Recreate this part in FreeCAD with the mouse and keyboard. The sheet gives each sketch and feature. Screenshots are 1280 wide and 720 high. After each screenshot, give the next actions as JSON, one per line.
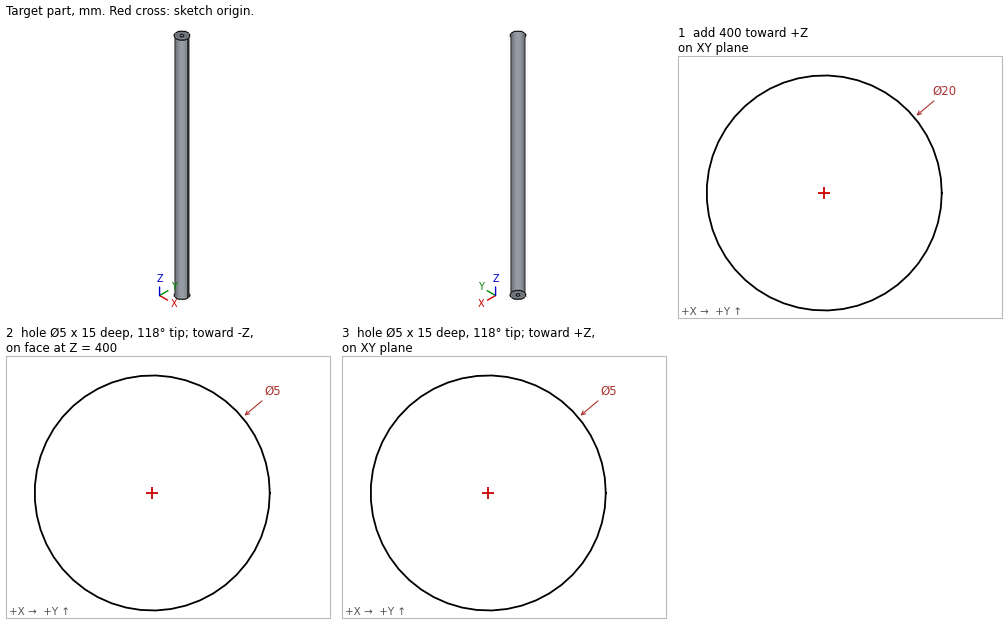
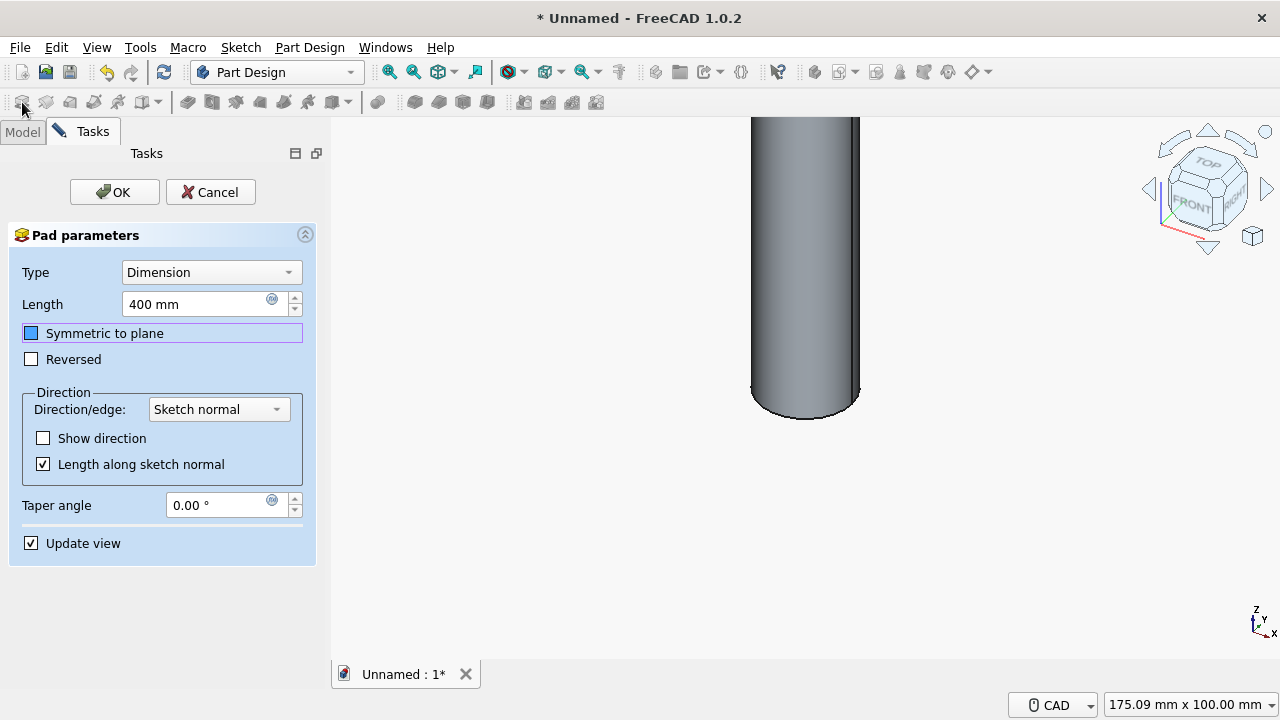
{"action": "left_click", "coordinate": [115, 192]}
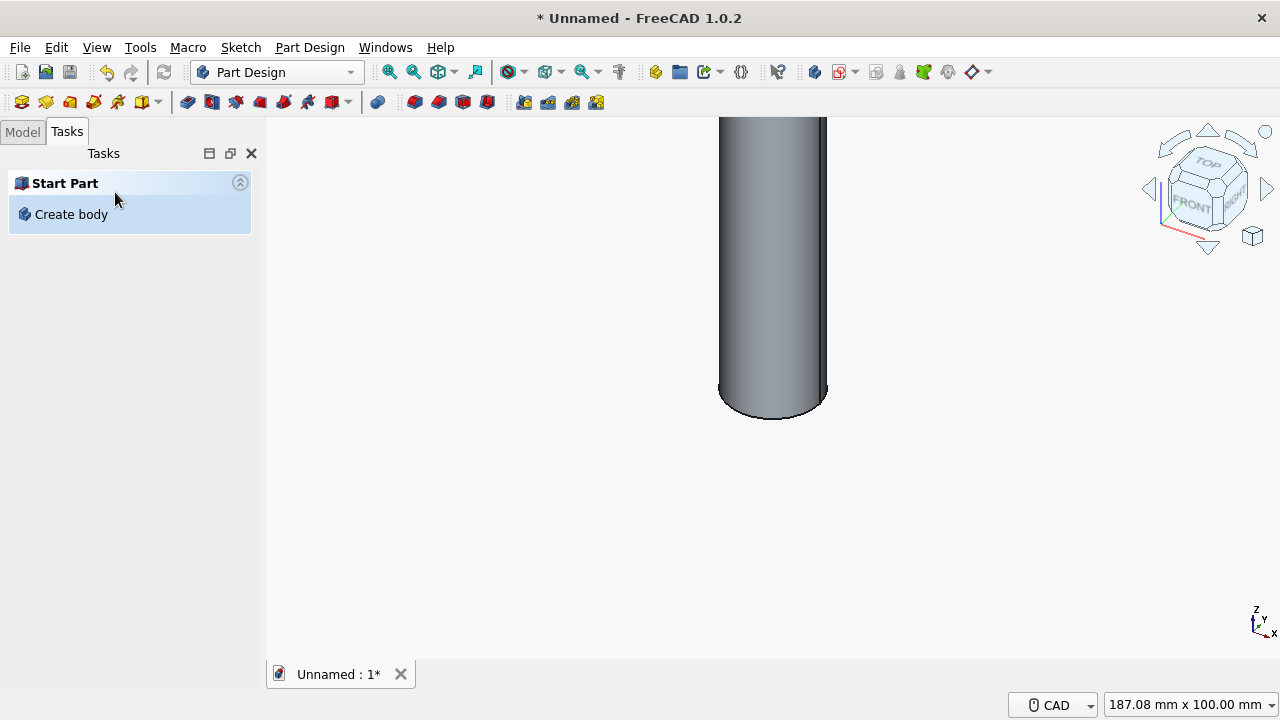
{"action": "key", "text": "v f"}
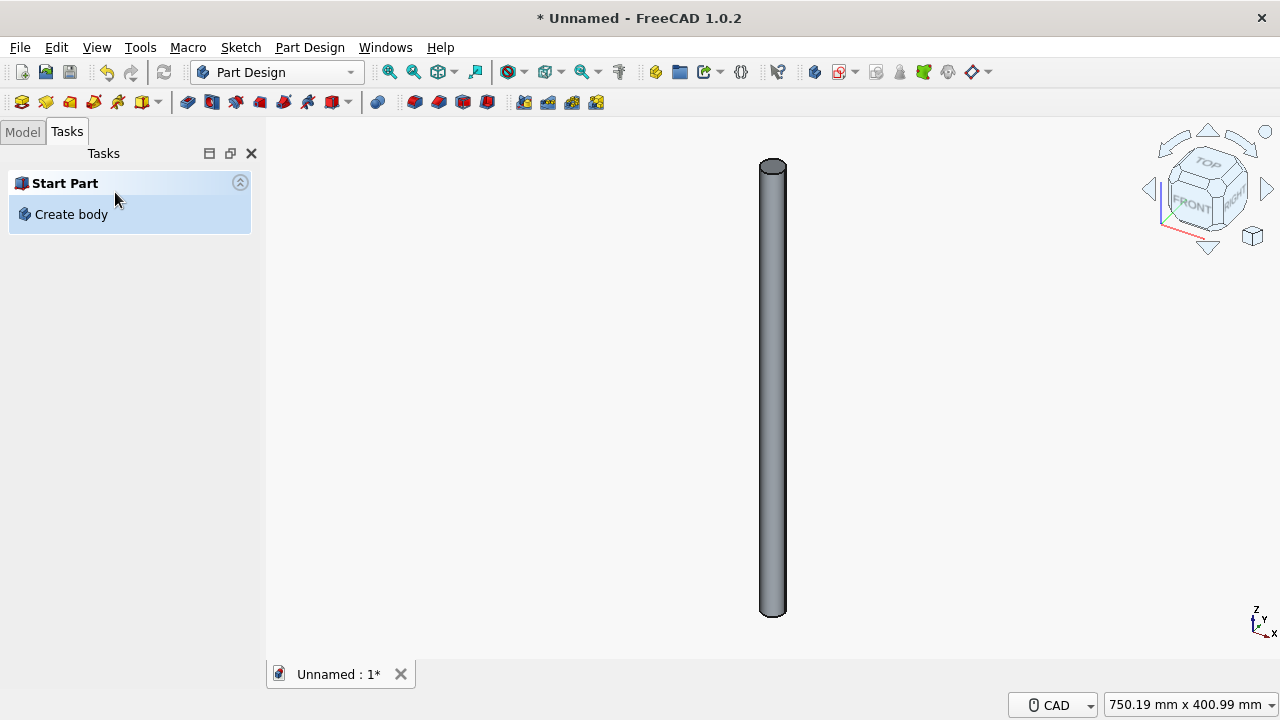
{"action": "left_click", "coordinate": [770, 164]}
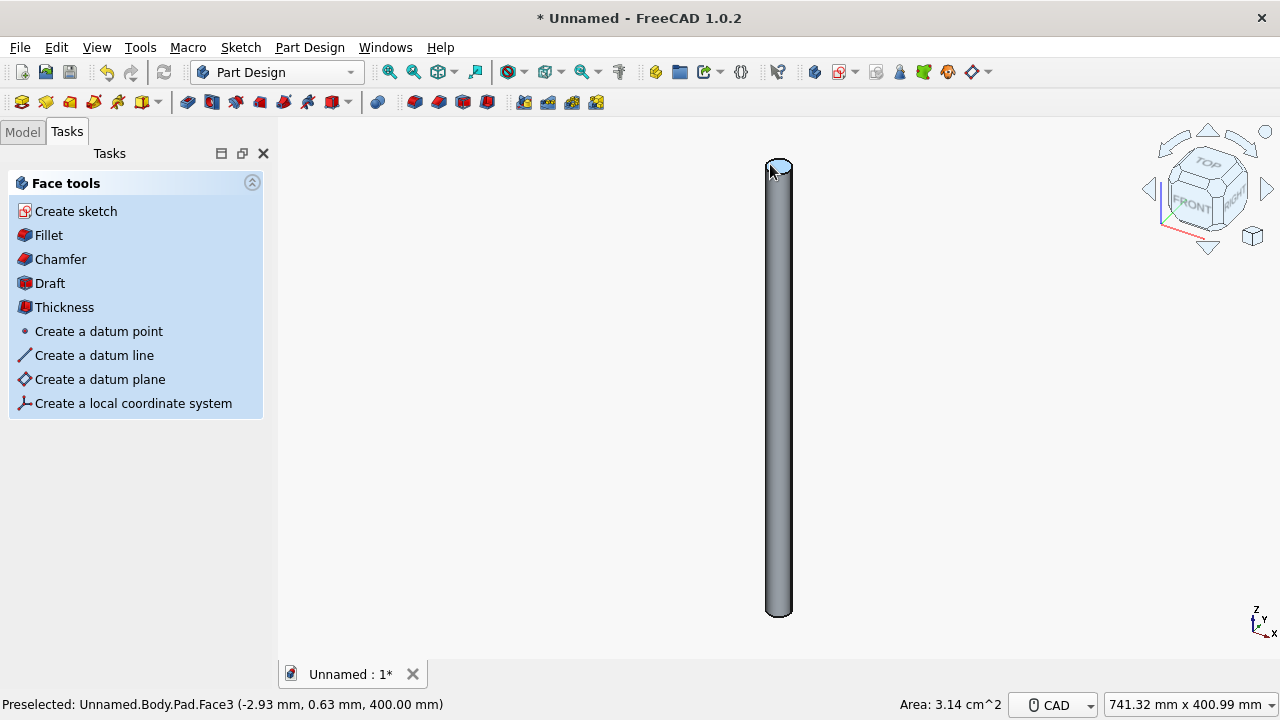
{"action": "left_click", "coordinate": [840, 72]}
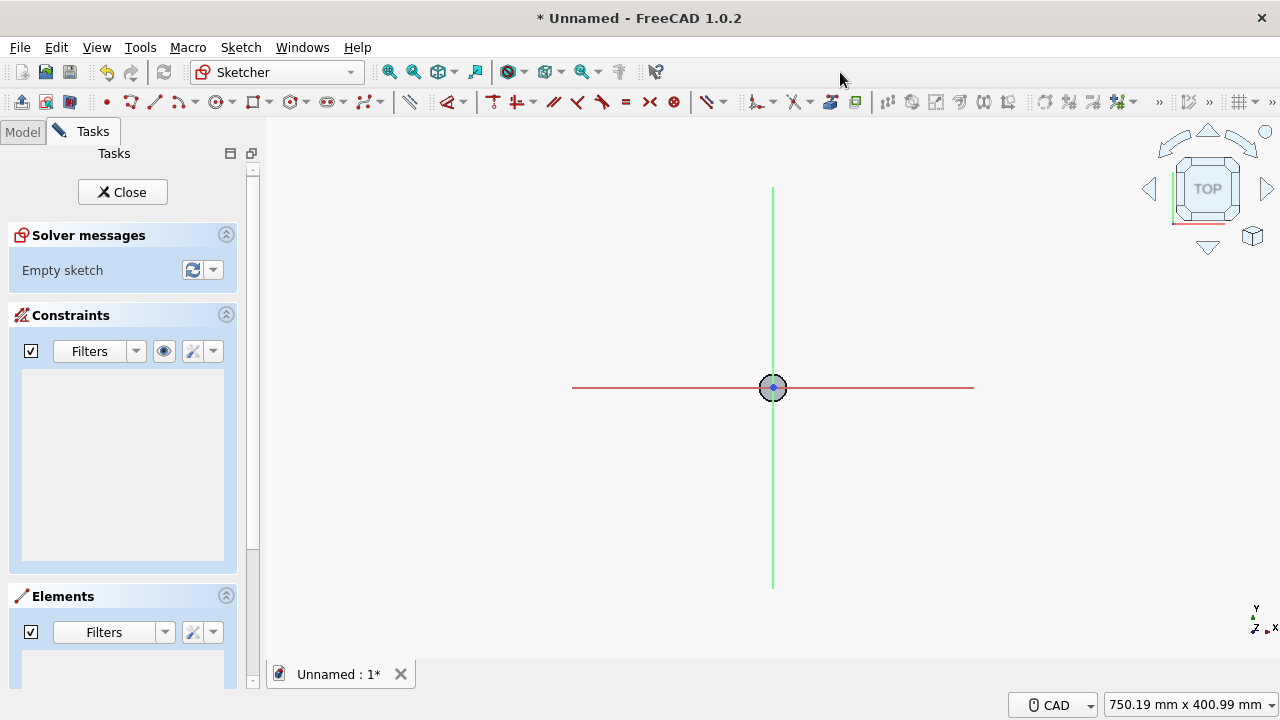
{"action": "scroll", "coordinate": [777, 388], "scroll_direction": "up", "scroll_amount": 15}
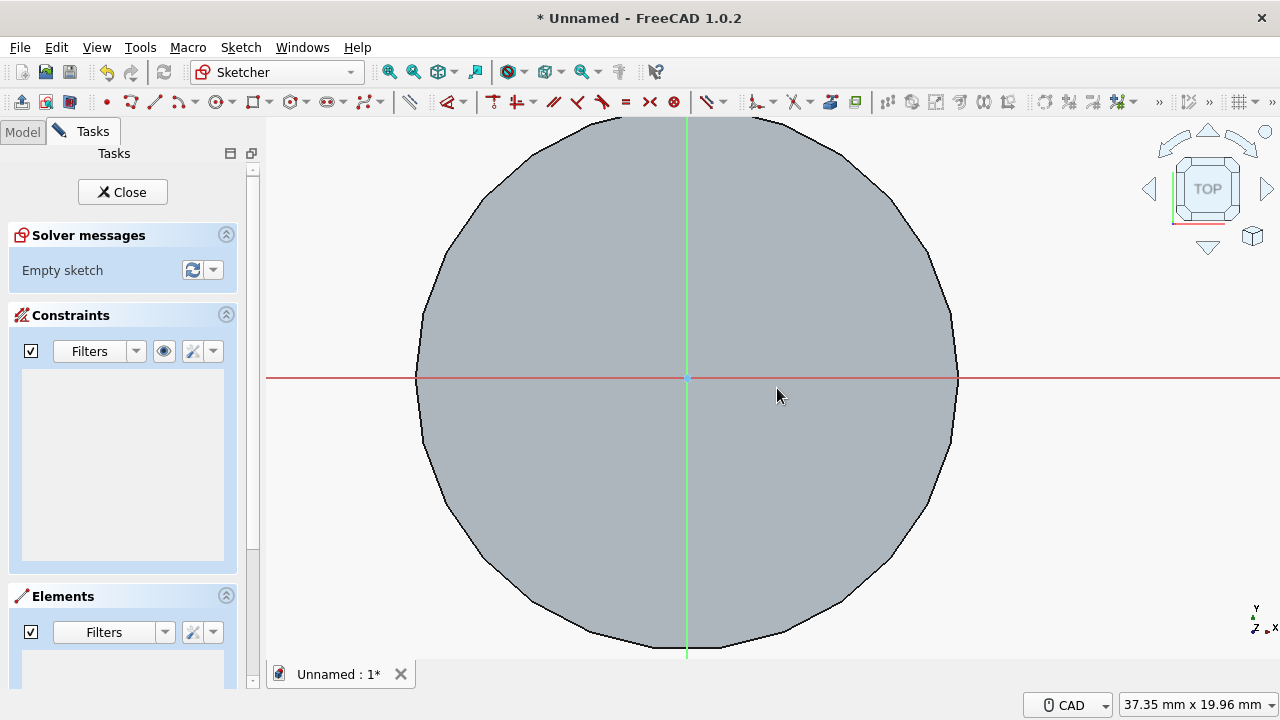
{"action": "scroll", "coordinate": [677, 373], "scroll_direction": "up", "scroll_amount": 5}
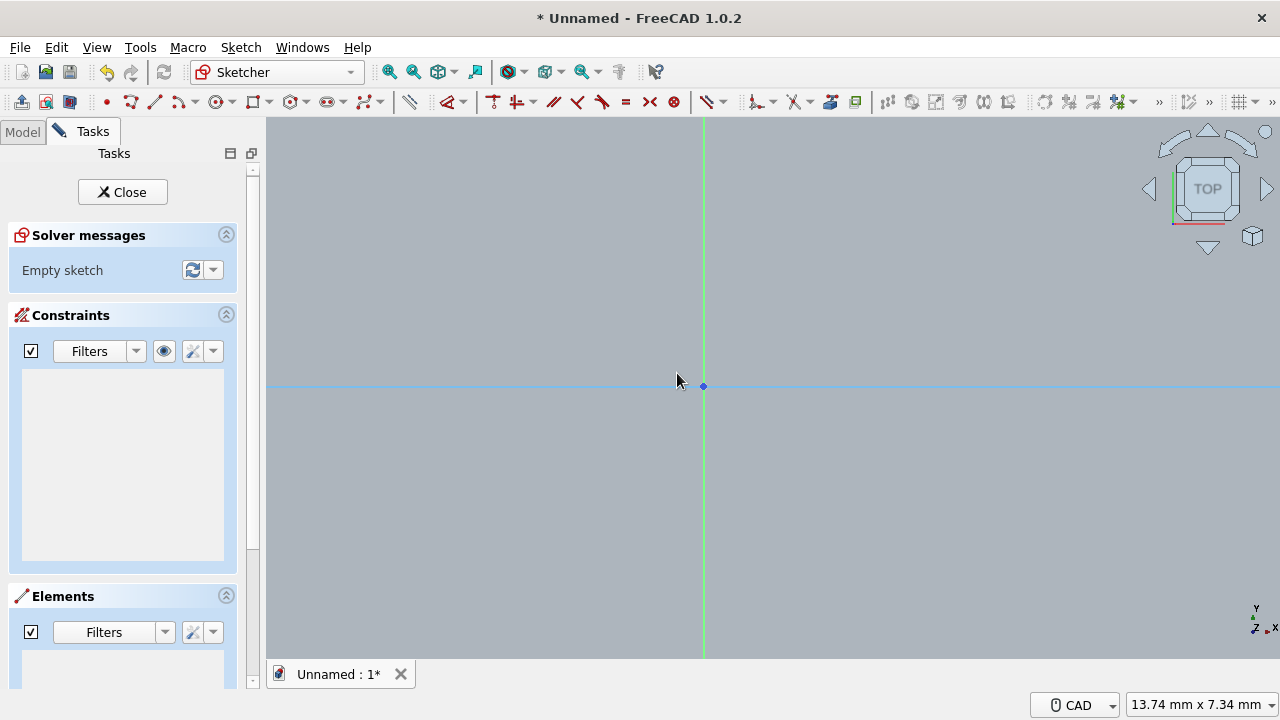
{"action": "left_click", "coordinate": [216, 102]}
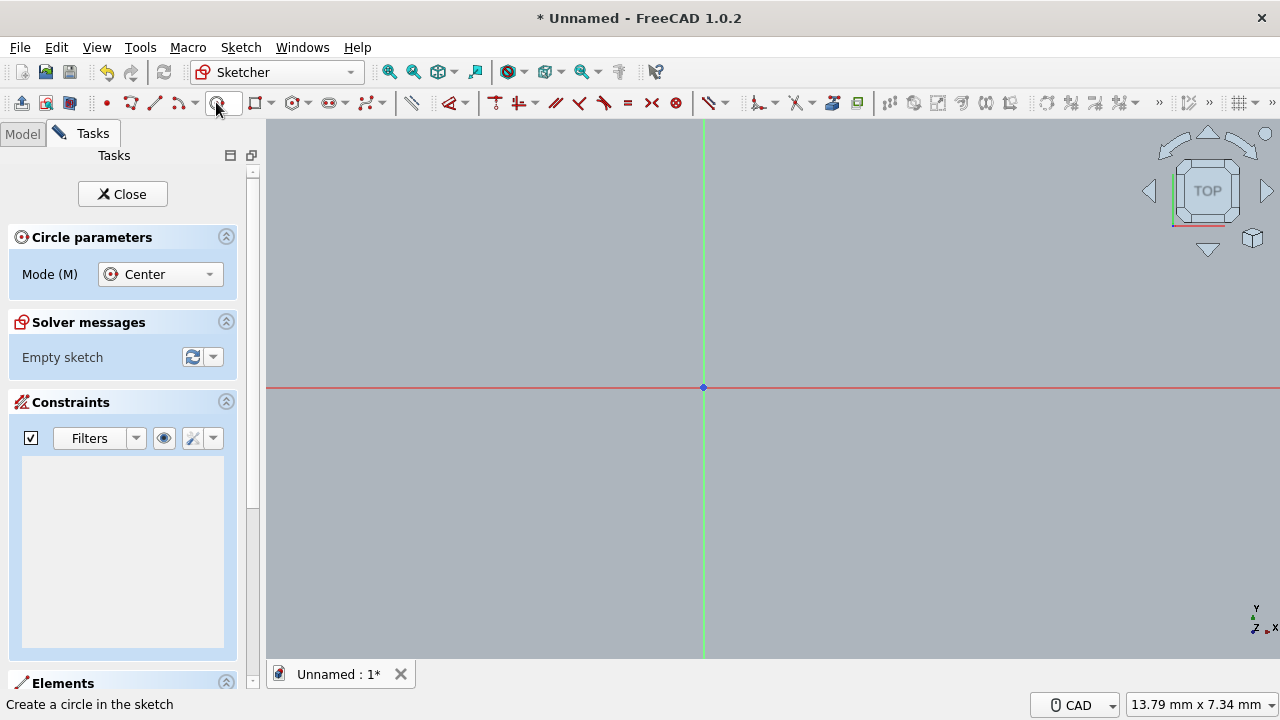
{"action": "left_click", "coordinate": [704, 388]}
{"action": "mouse_move", "coordinate": [834, 258]}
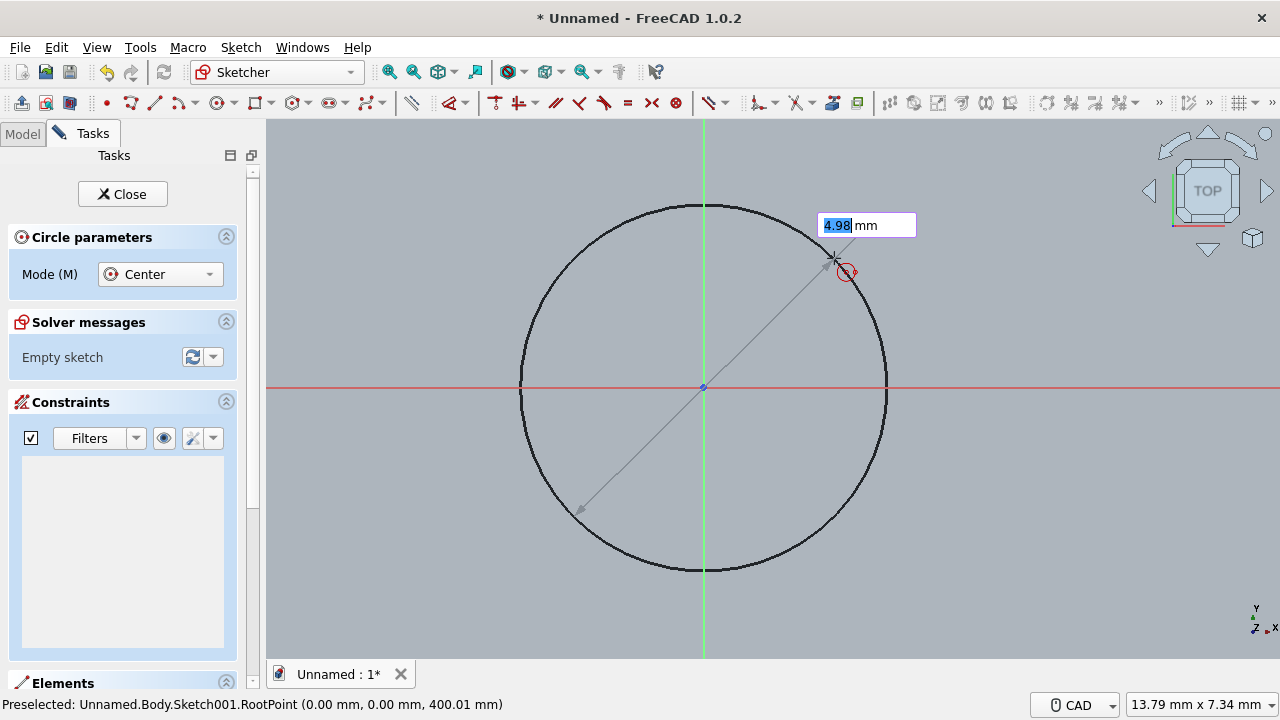
{"action": "type", "text": "5"}
{"action": "key", "text": "Return"}
{"action": "key", "text": "Escape"}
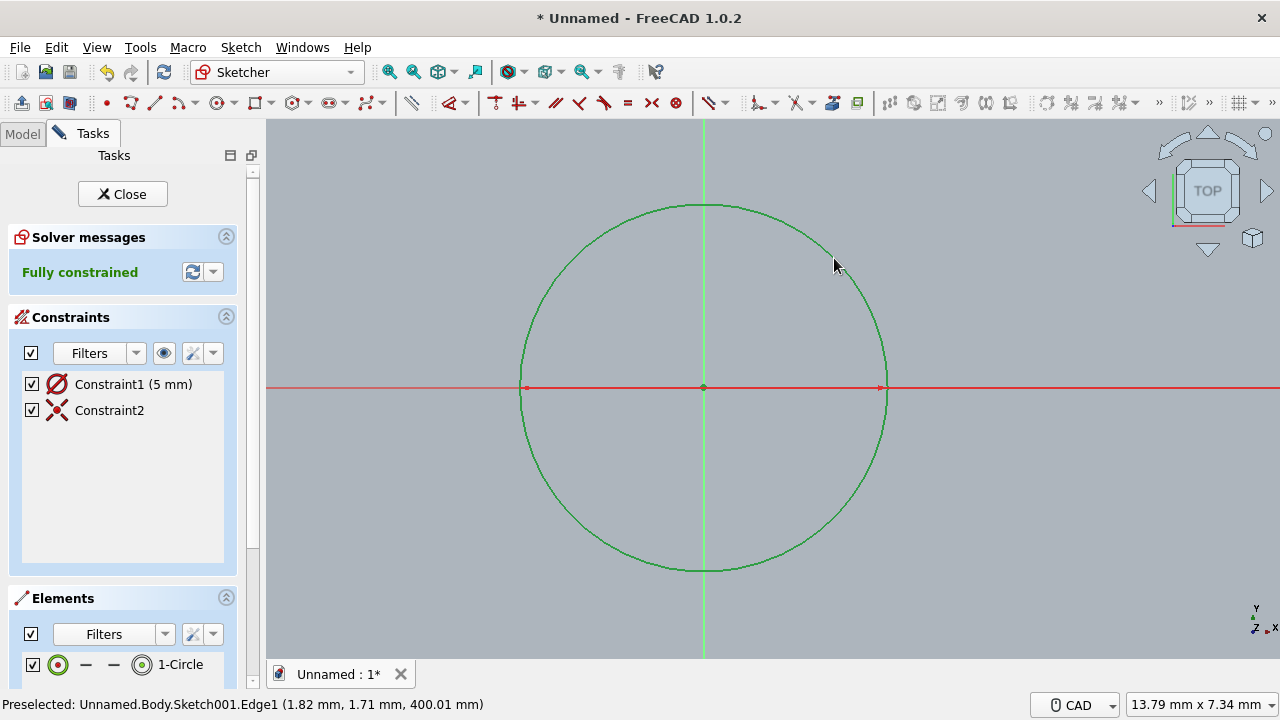
{"action": "left_click", "coordinate": [123, 194]}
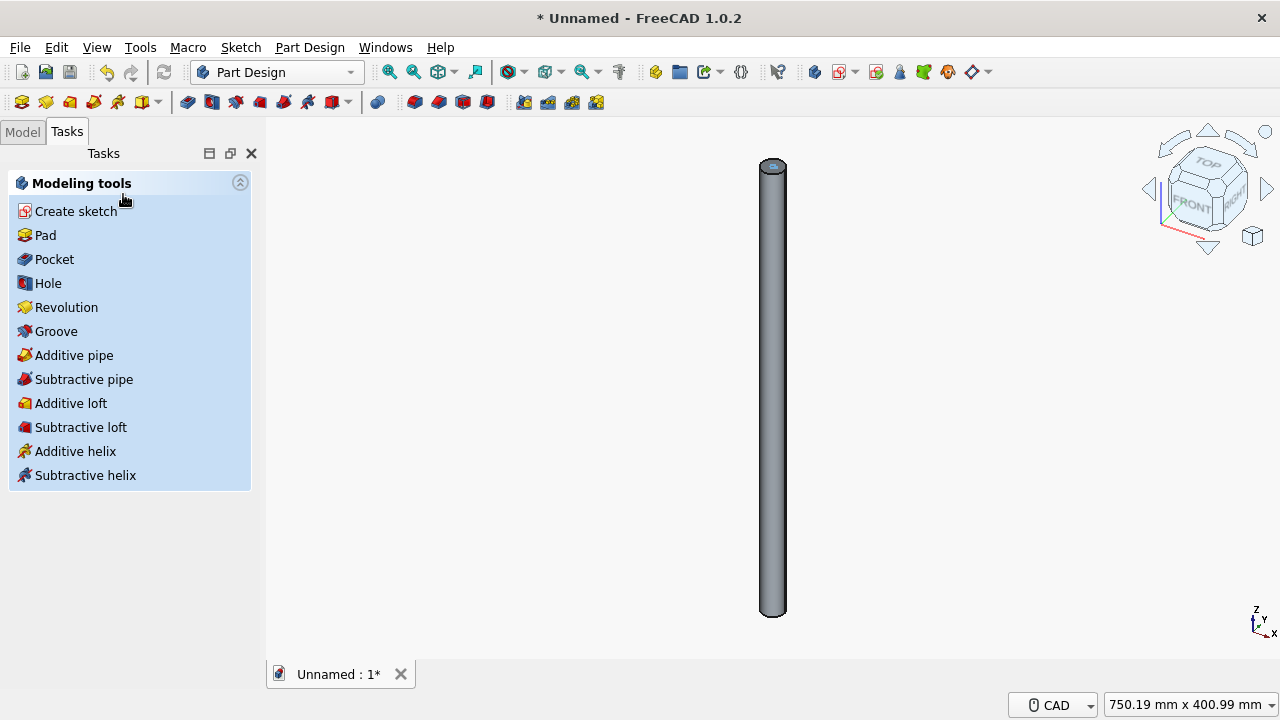
{"action": "left_click", "coordinate": [212, 102]}